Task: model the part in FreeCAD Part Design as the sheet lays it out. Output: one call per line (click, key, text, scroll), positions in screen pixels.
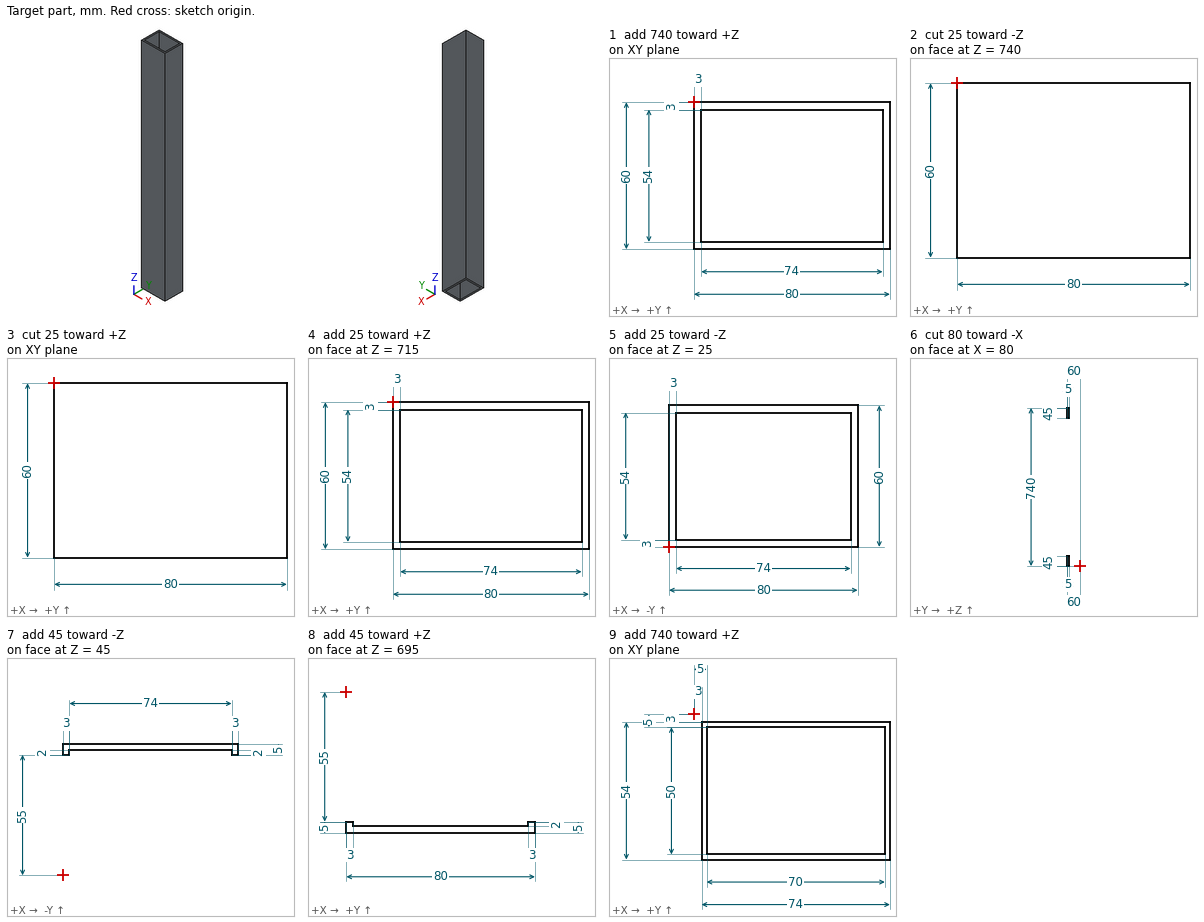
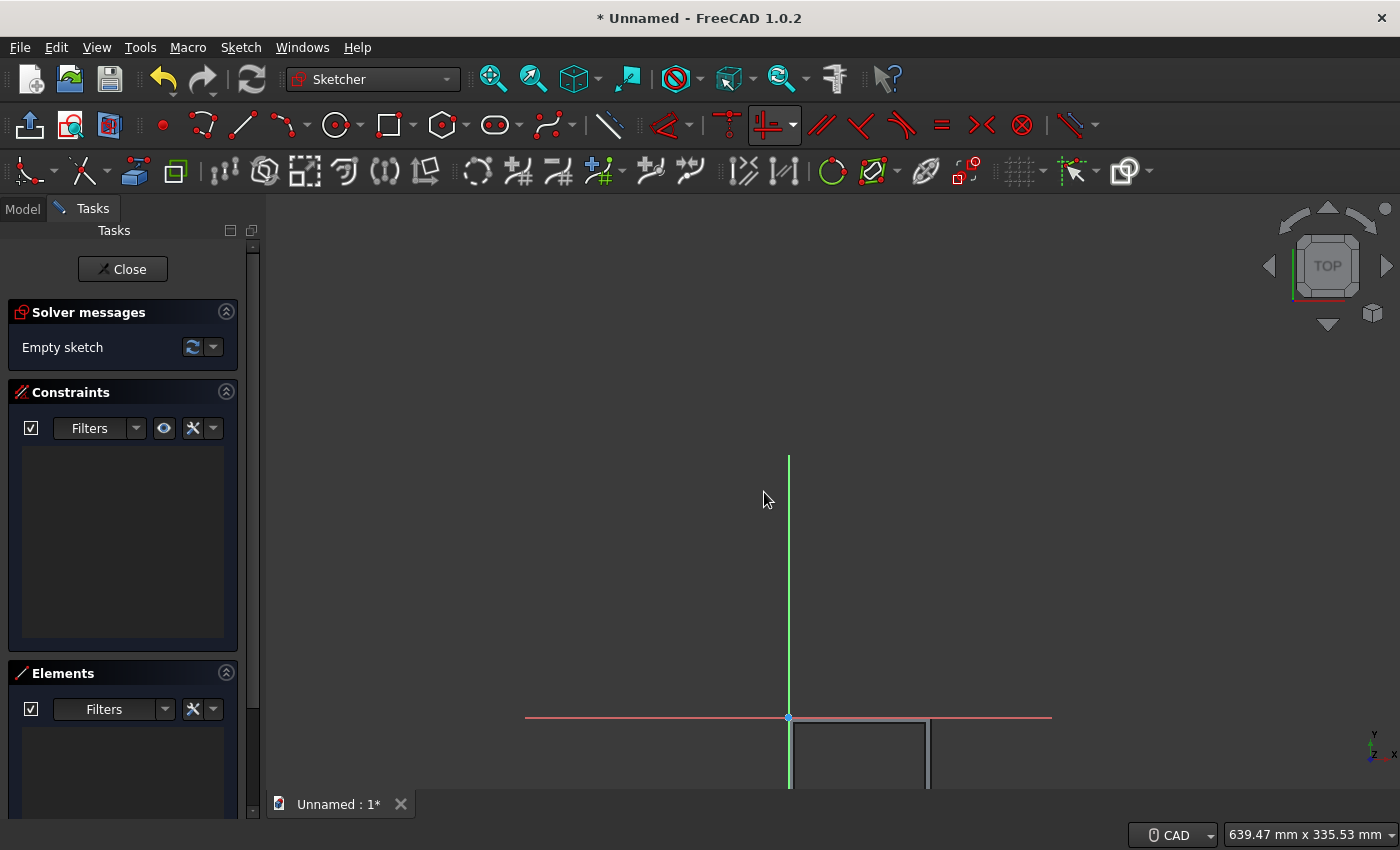
scroll(764, 492, down, 5)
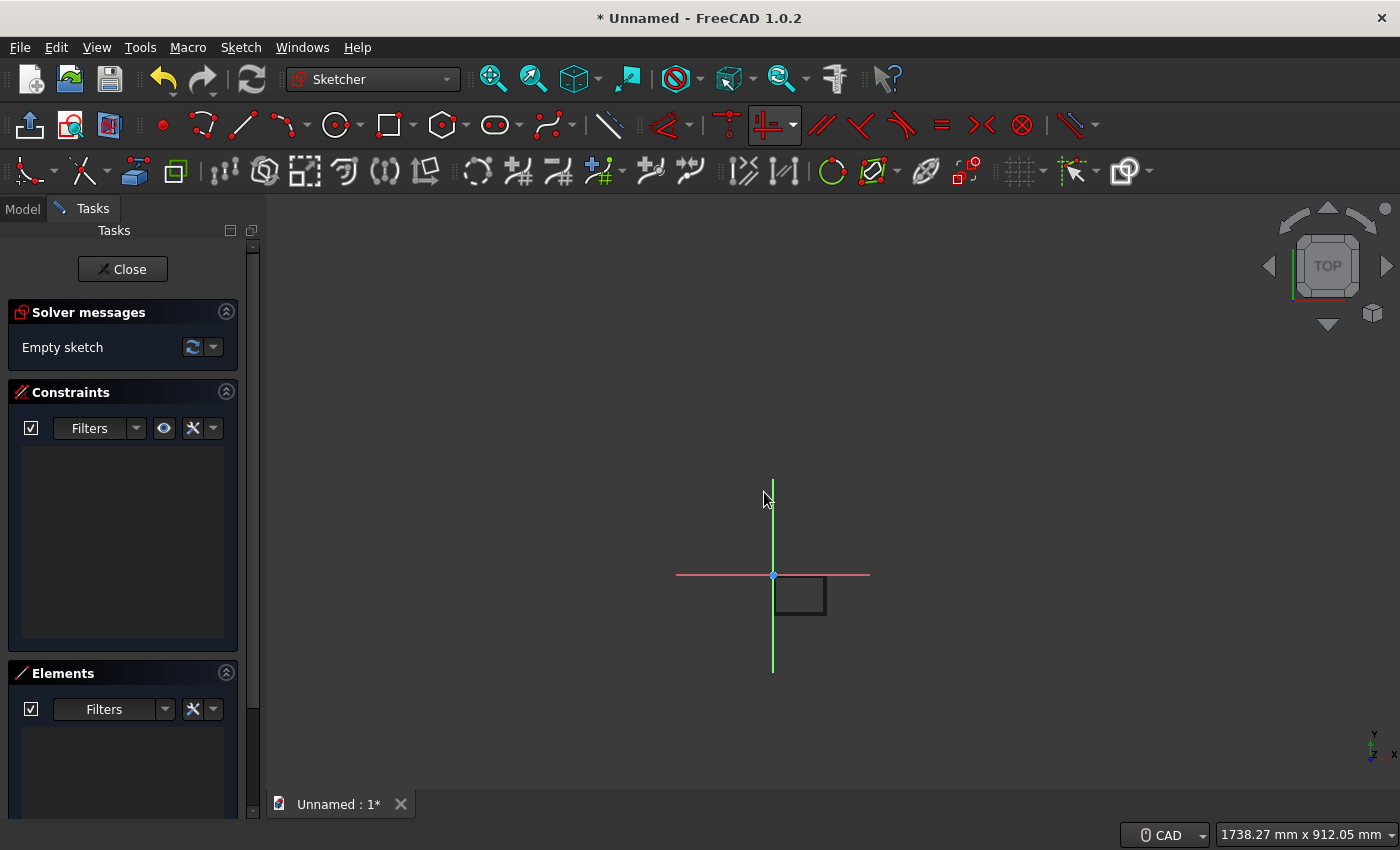
scroll(804, 608, up, 11)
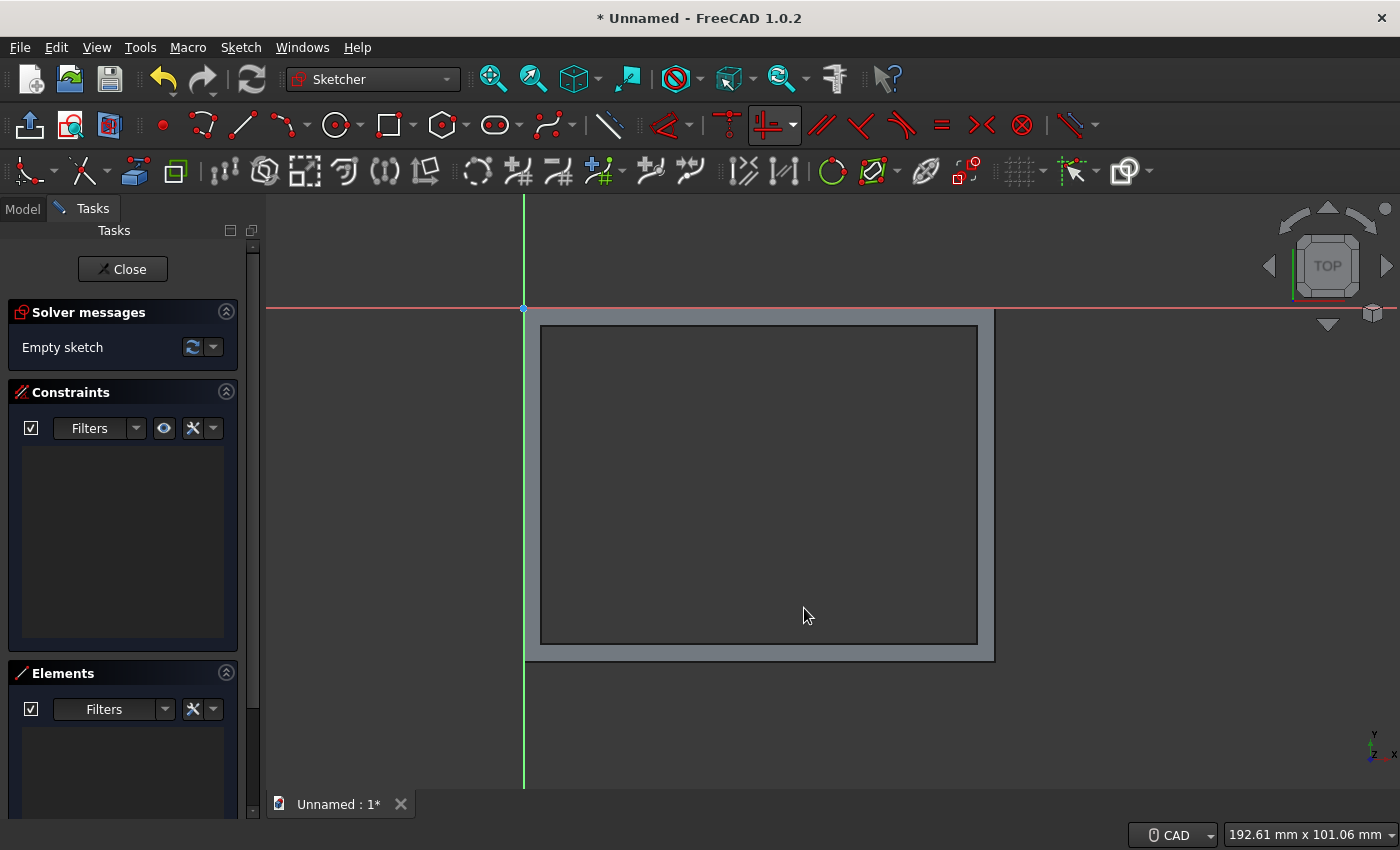
key(g)
key(r)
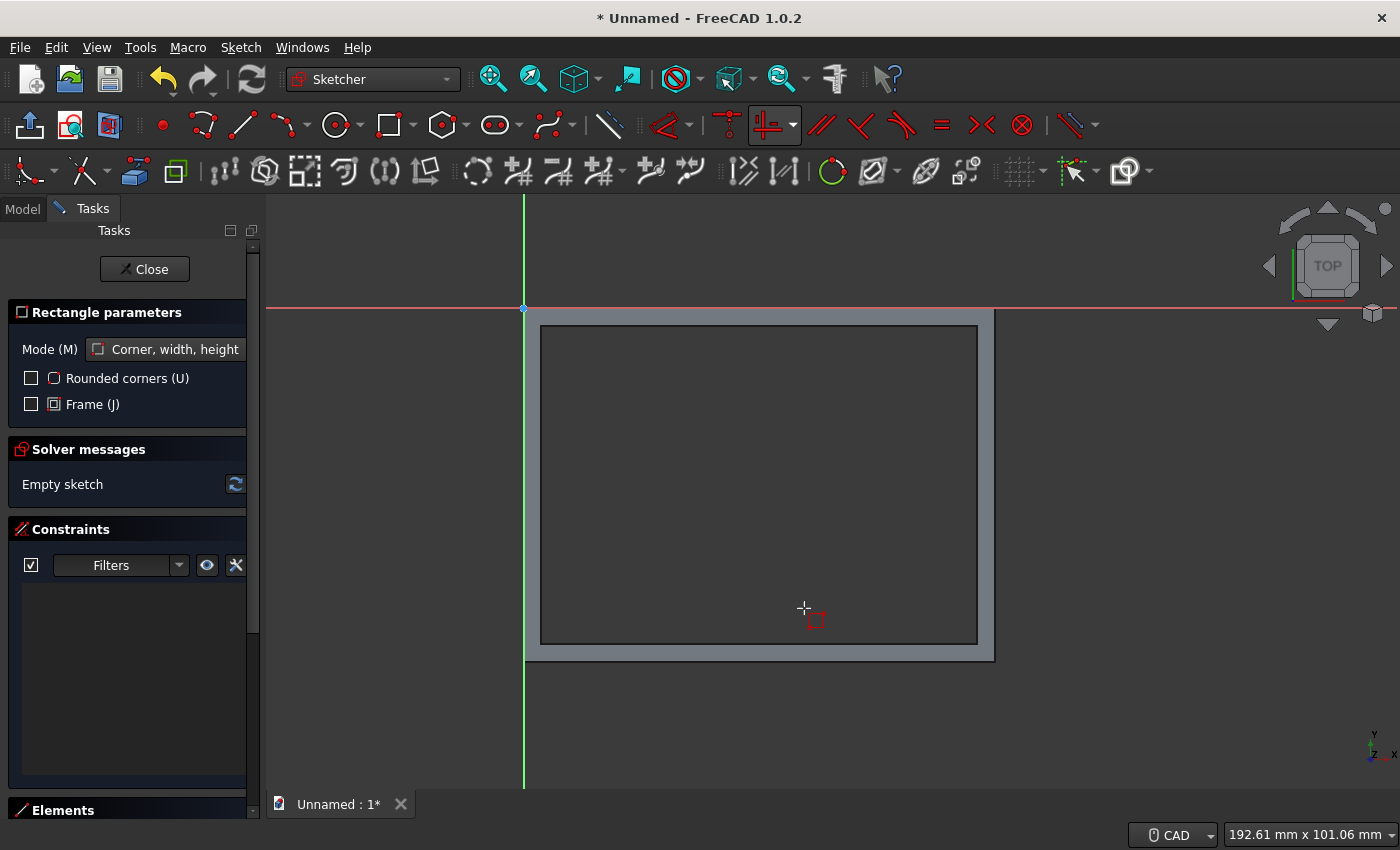
click(524, 308)
click(995, 662)
key(Escape)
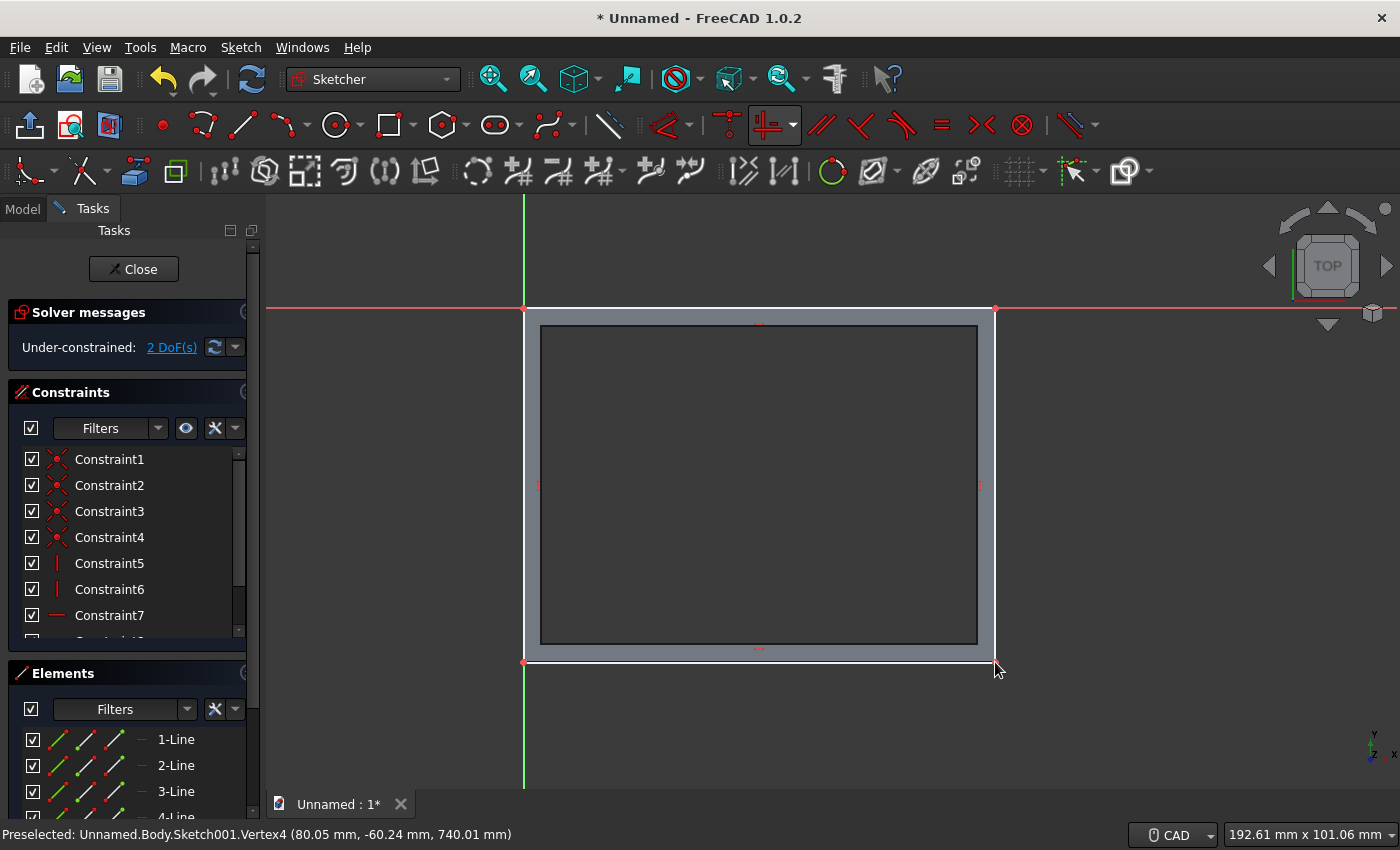
key(d)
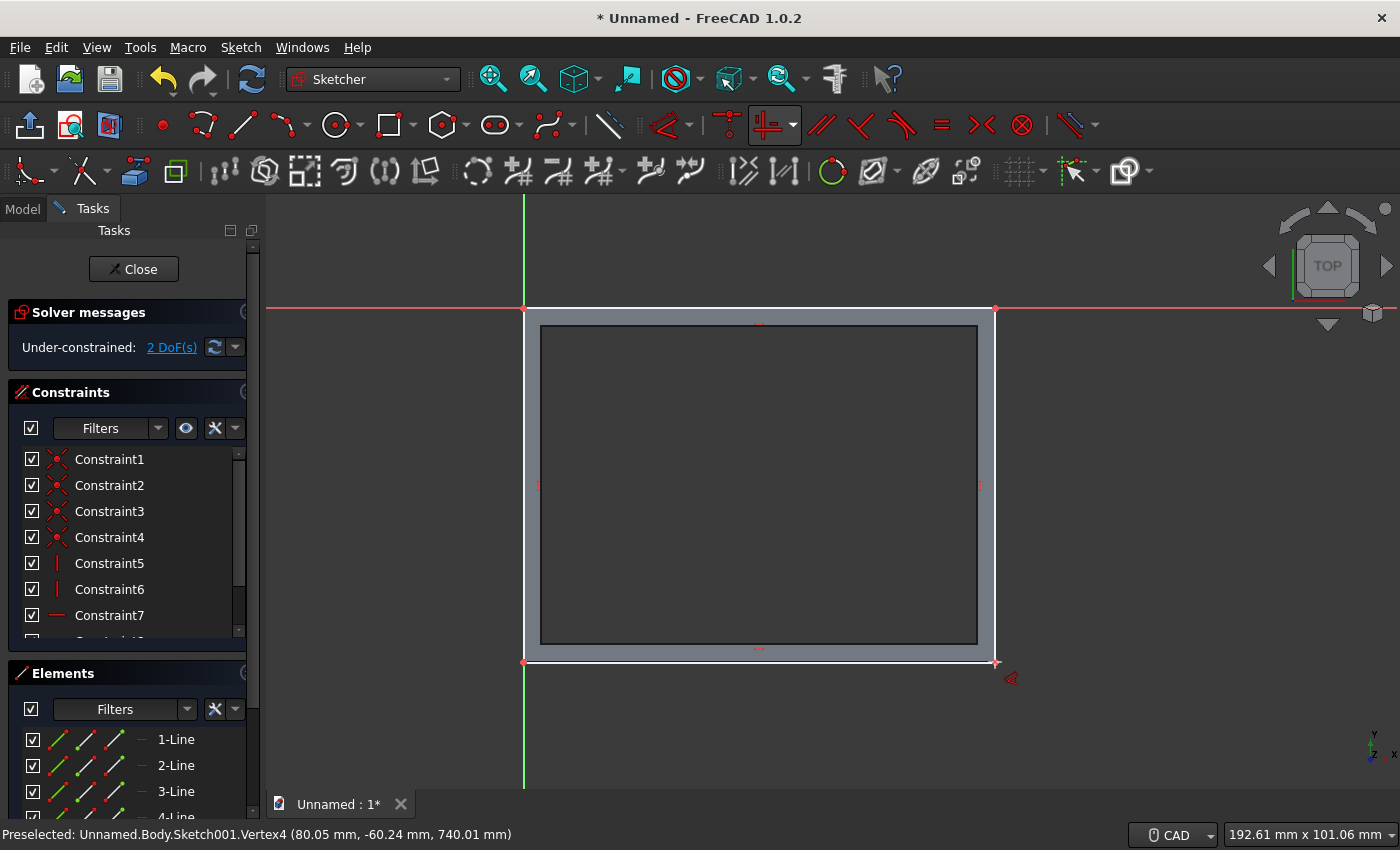
click(524, 415)
click(490, 486)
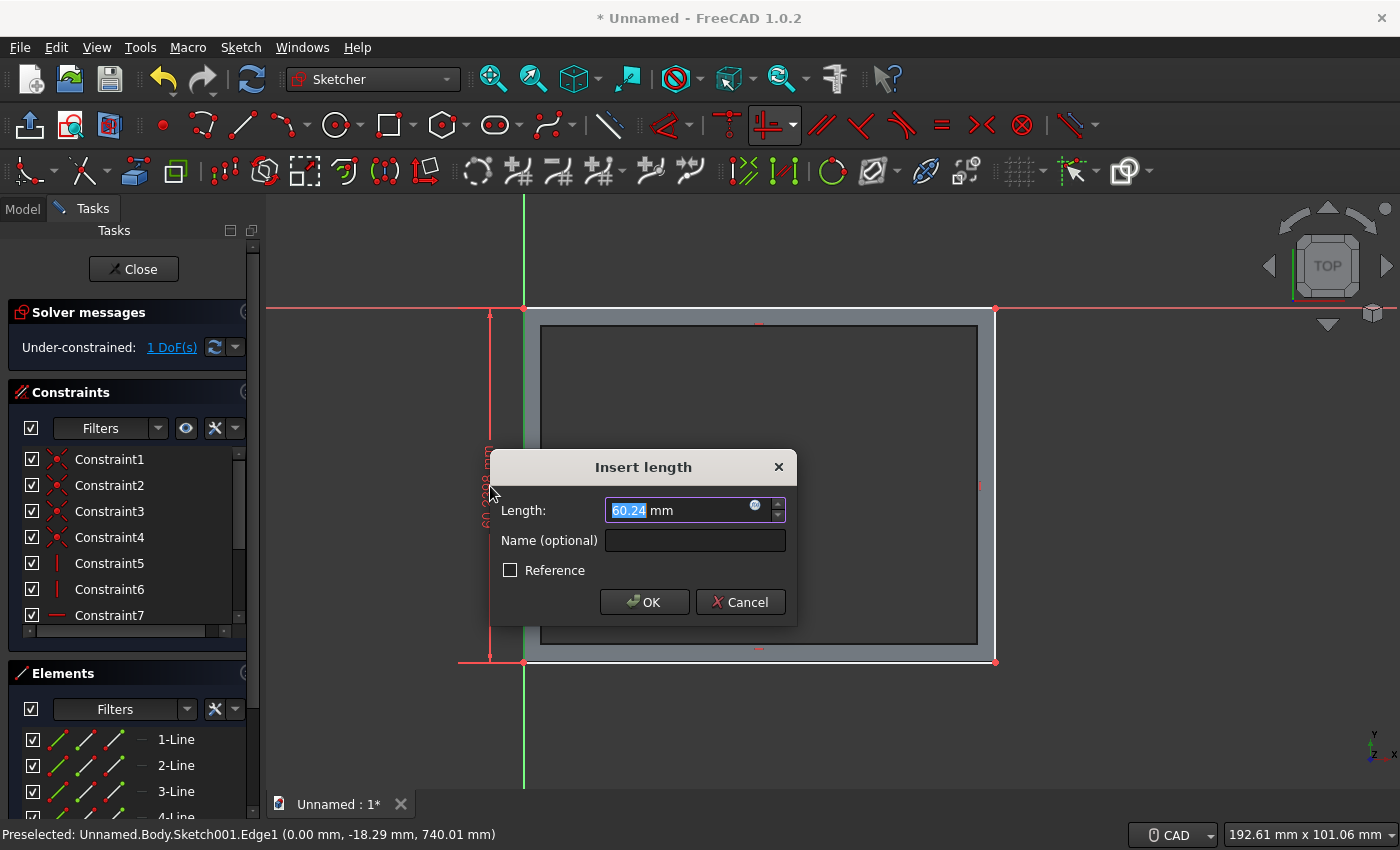
text(60)
key(Return)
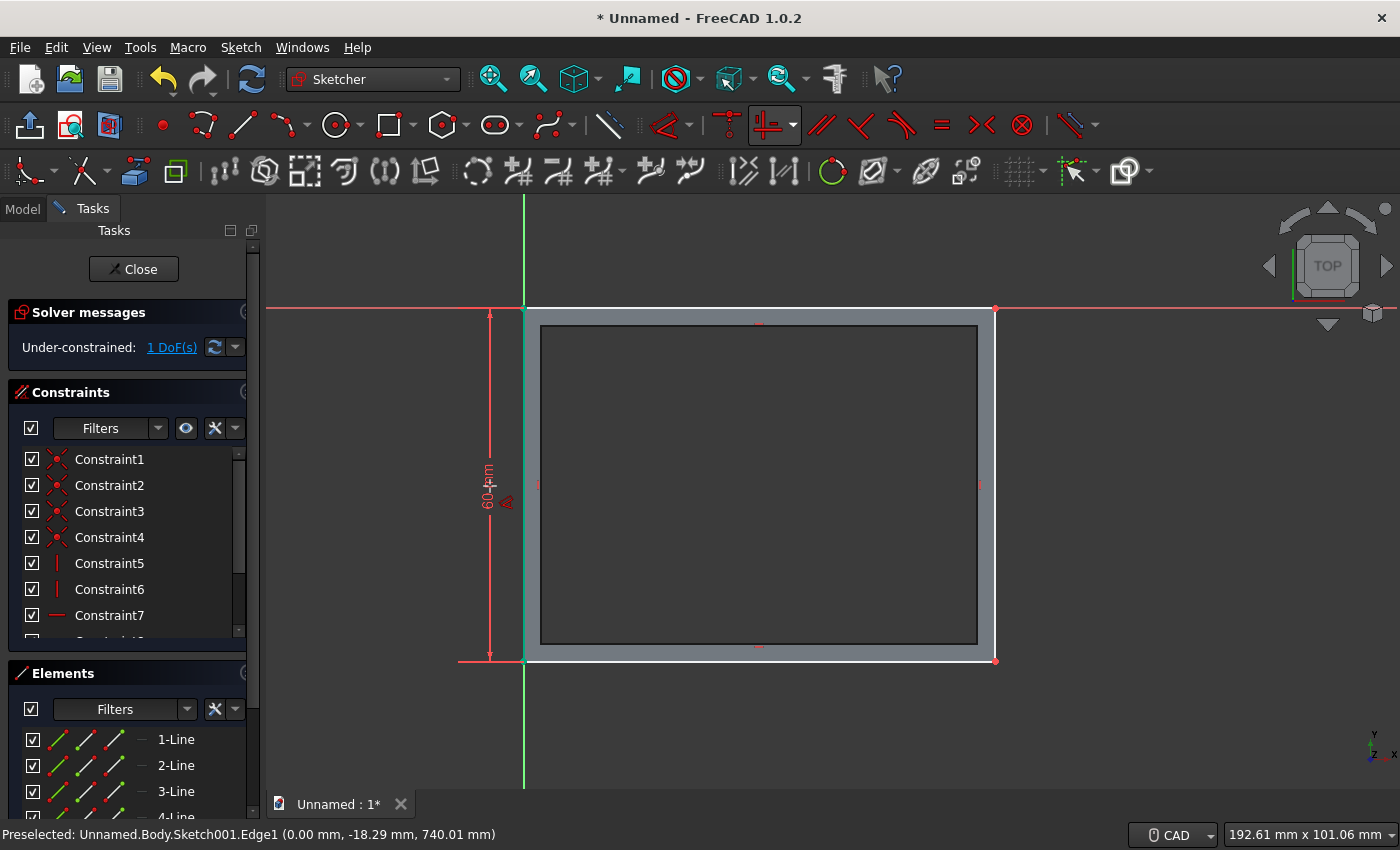
click(665, 662)
click(759, 696)